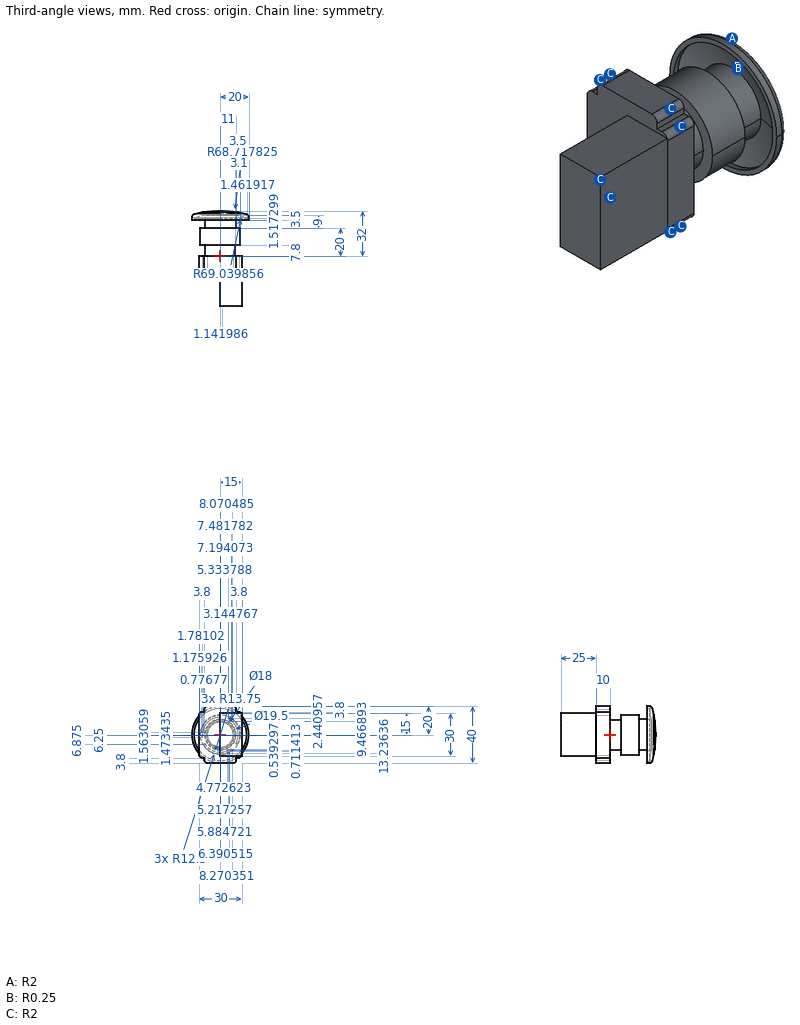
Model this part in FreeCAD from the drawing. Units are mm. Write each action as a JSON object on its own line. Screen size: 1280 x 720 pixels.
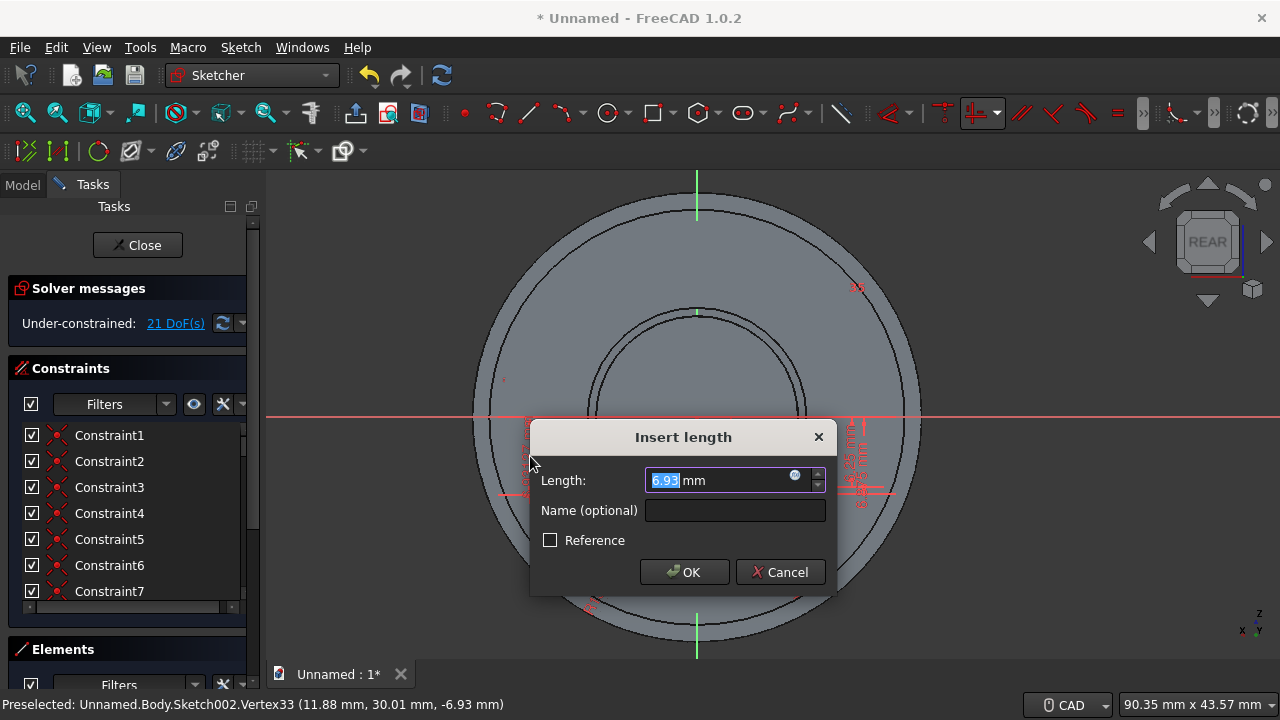
{"action": "type", "text": "6.875"}
{"action": "key", "text": "Return"}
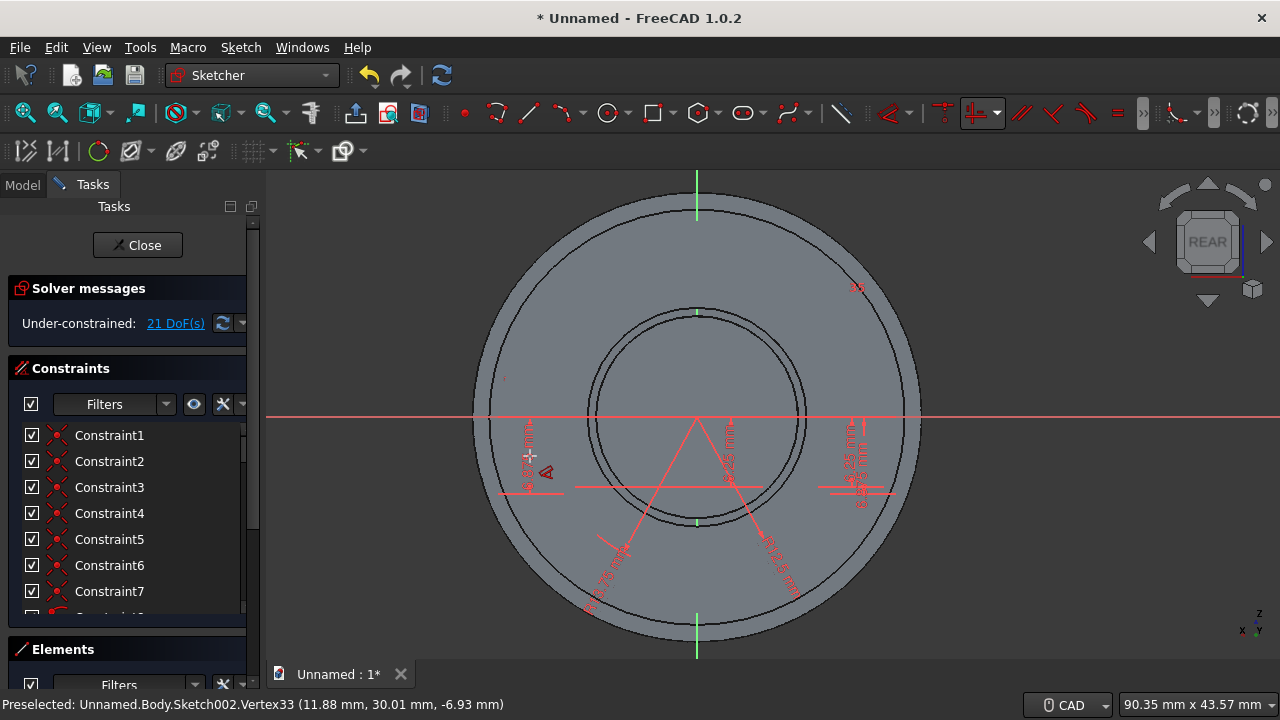
{"action": "scroll", "coordinate": [832, 401], "scroll_direction": "up", "scroll_amount": 8}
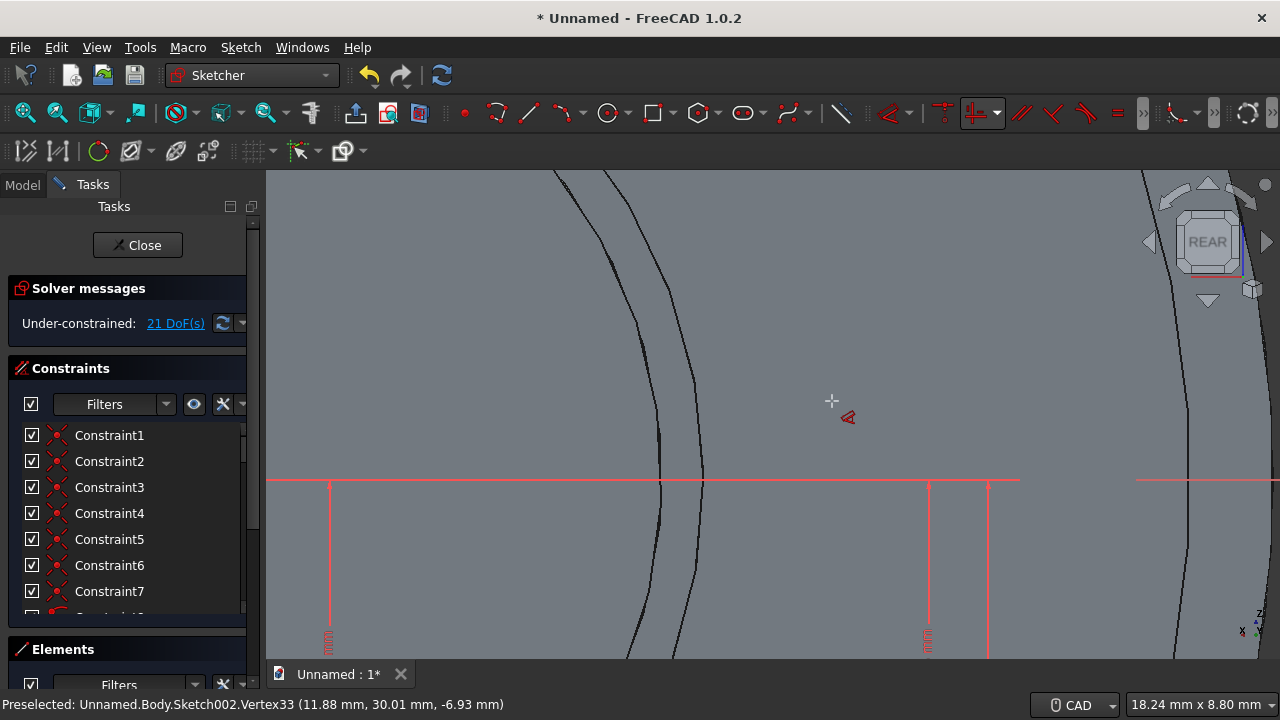
{"action": "left_click", "coordinate": [829, 397]}
{"action": "left_click", "coordinate": [829, 363]}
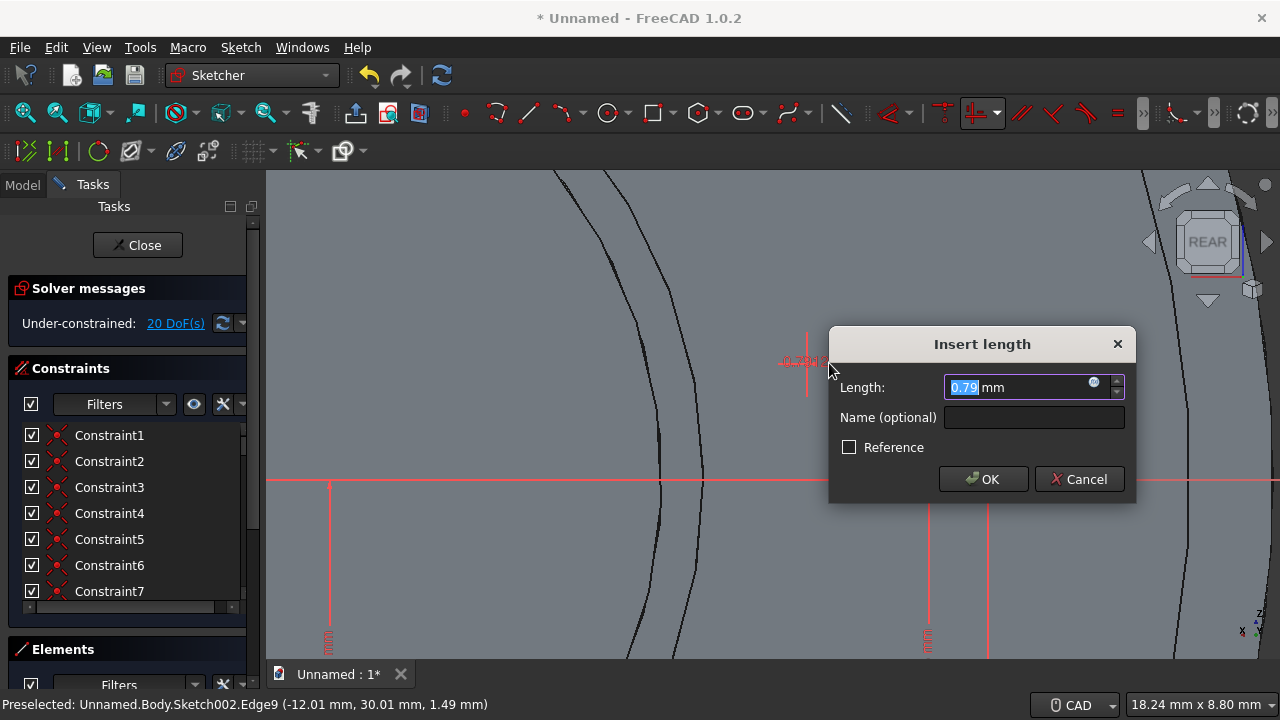
{"action": "type", "text": "0.77677"}
{"action": "key", "text": "Return"}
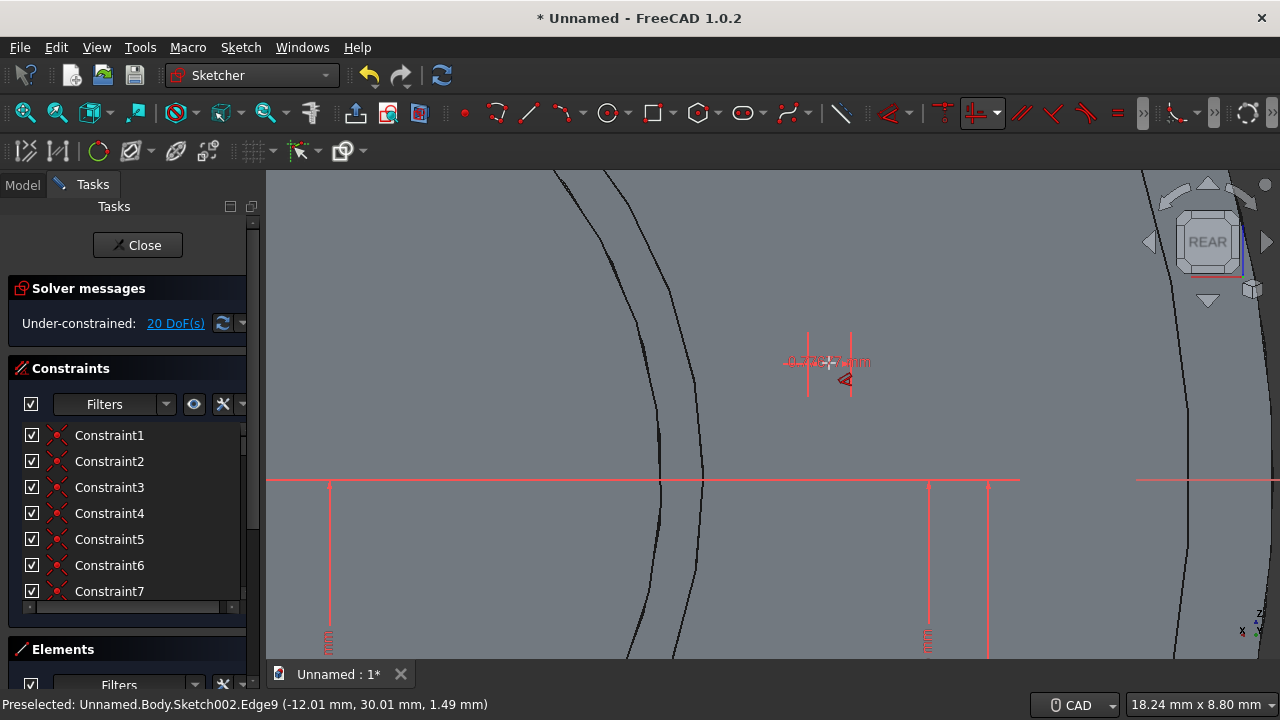
{"action": "left_click", "coordinate": [967, 396]}
{"action": "left_click", "coordinate": [954, 362]}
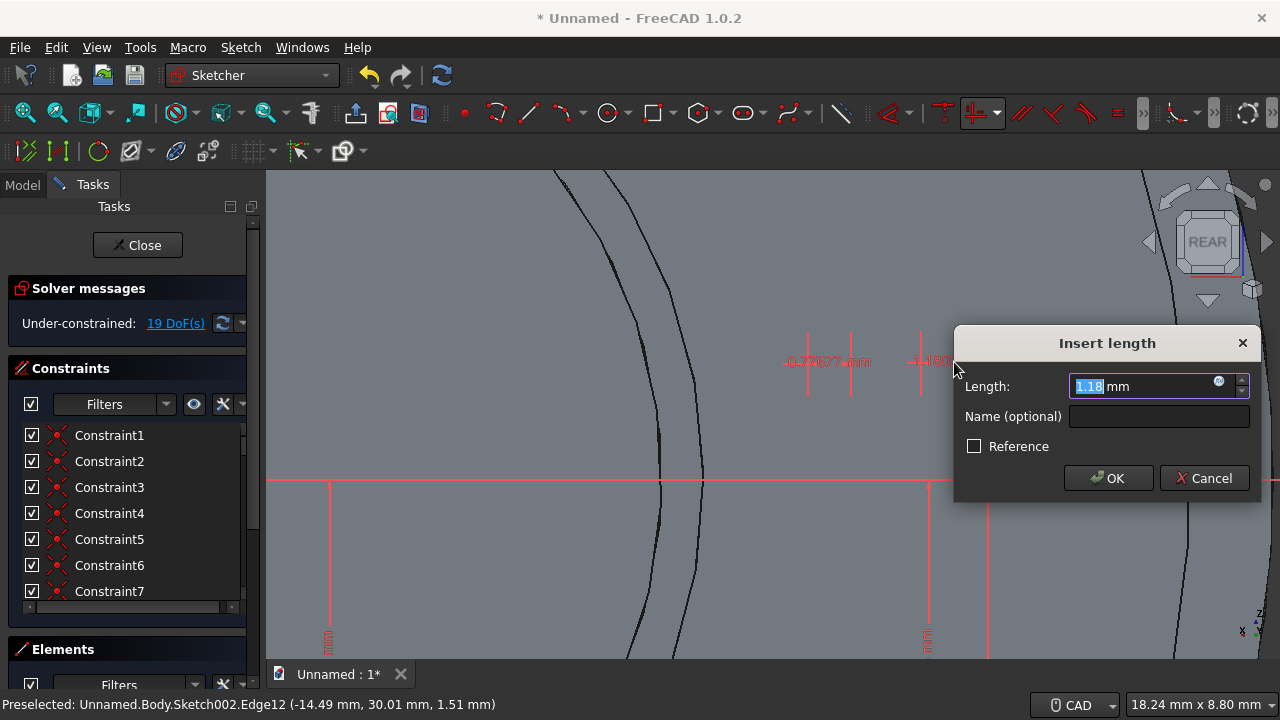
{"action": "type", "text": "1.175926"}
{"action": "key", "text": "Return"}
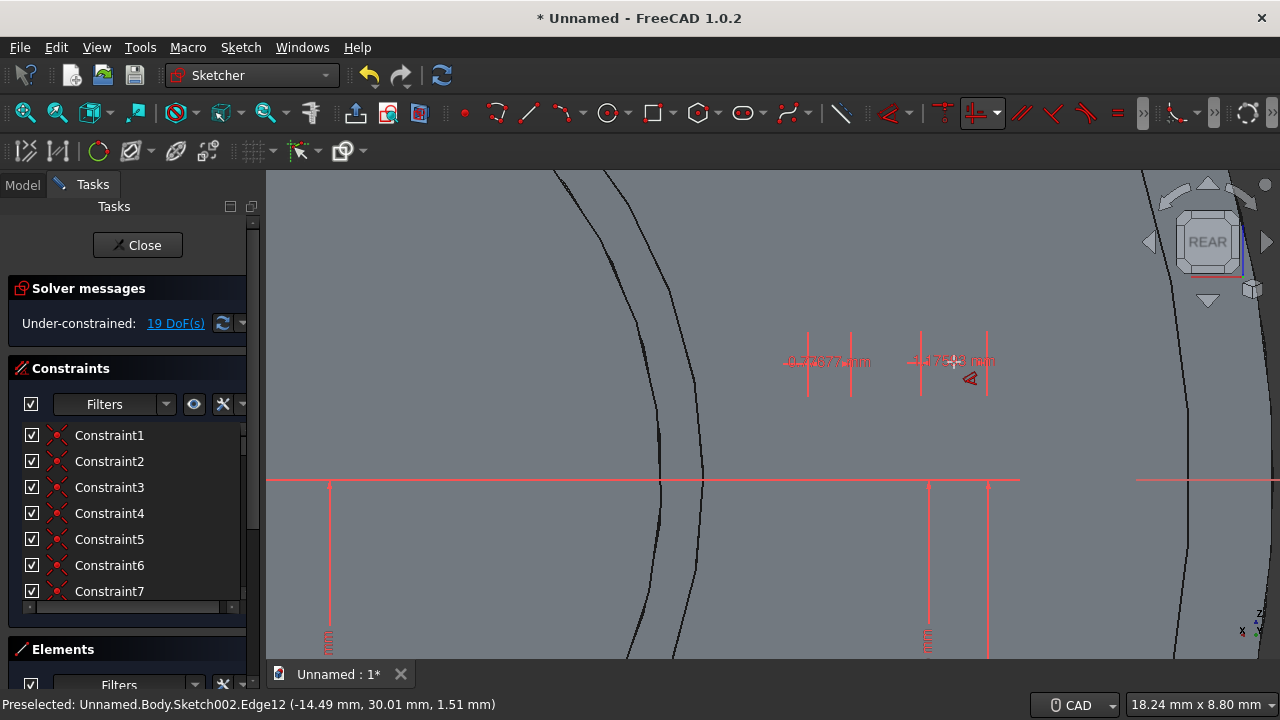
{"action": "scroll", "coordinate": [832, 402], "scroll_direction": "down", "scroll_amount": 8}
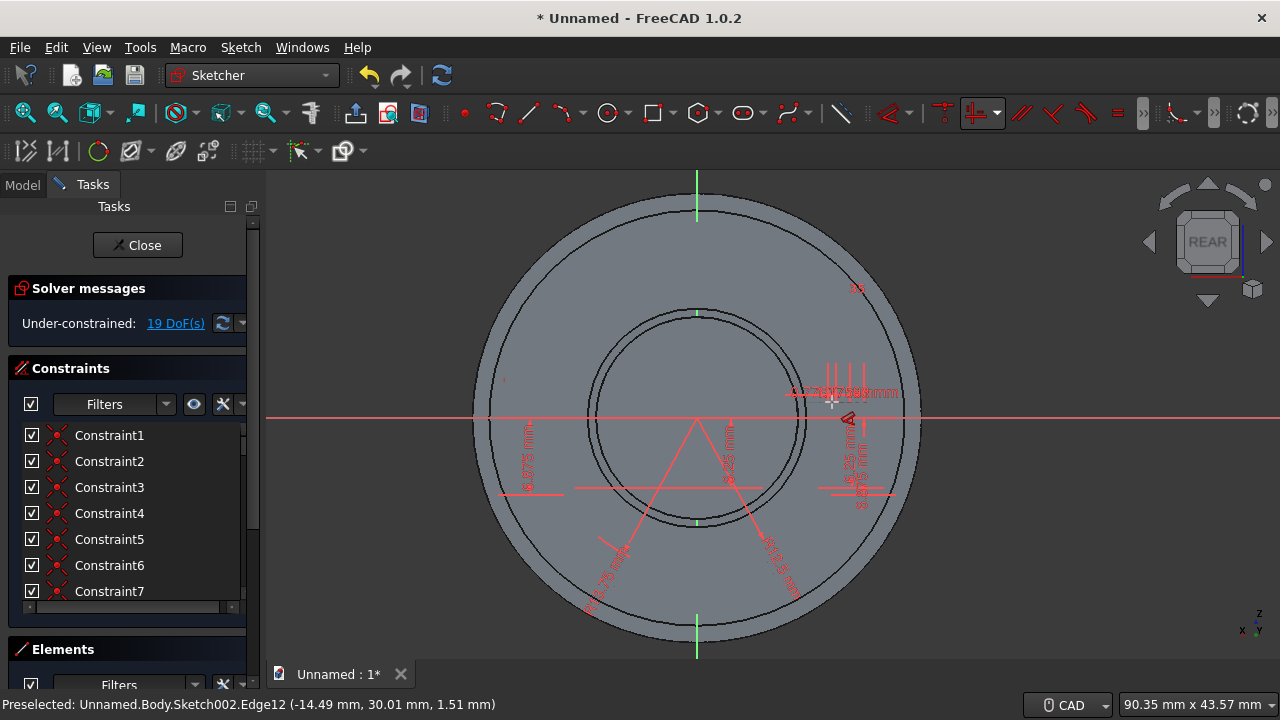
{"action": "scroll", "coordinate": [627, 285], "scroll_direction": "up", "scroll_amount": 3}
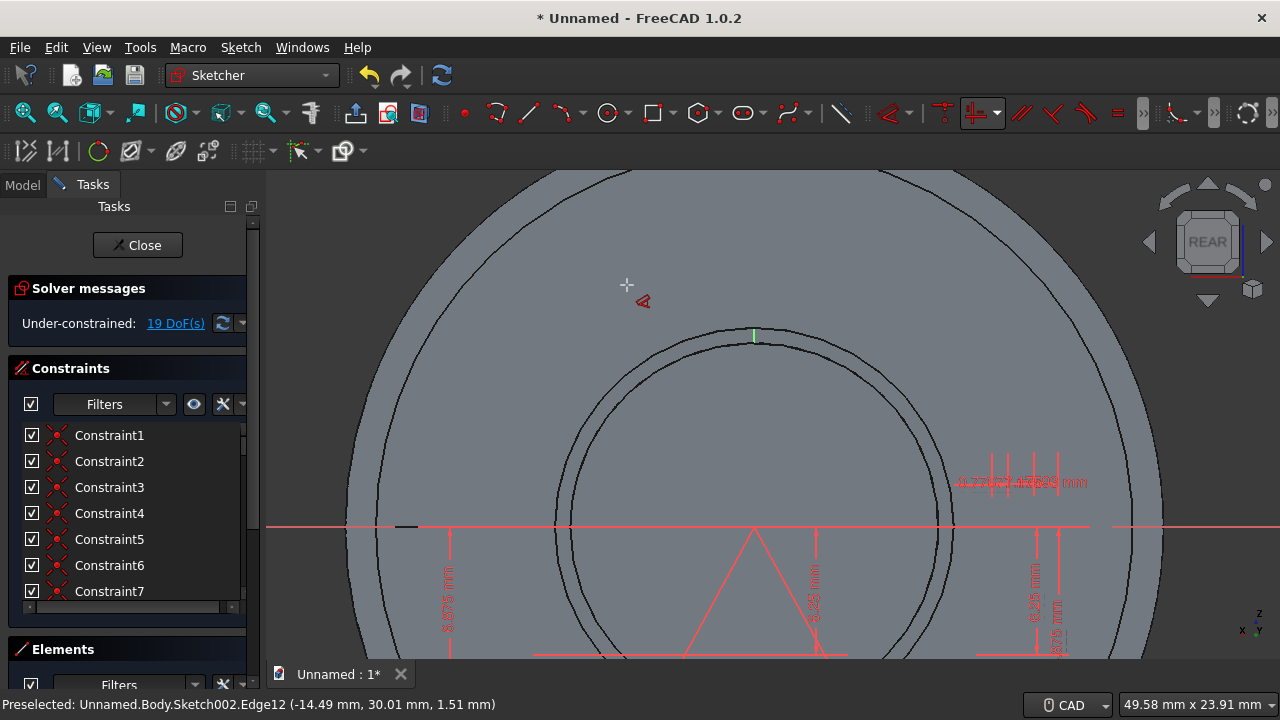
{"action": "left_click", "coordinate": [626, 284]}
{"action": "left_click", "coordinate": [613, 250]}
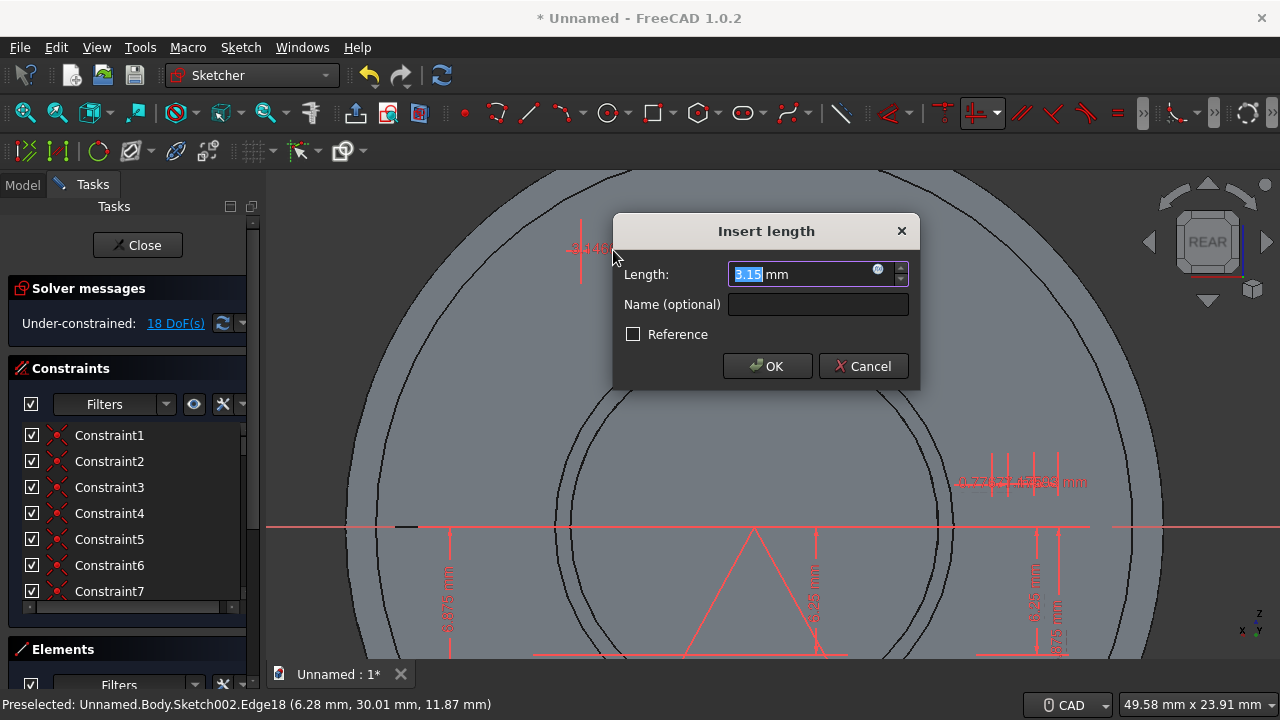
{"action": "type", "text": "3.144767"}
{"action": "key", "text": "Return"}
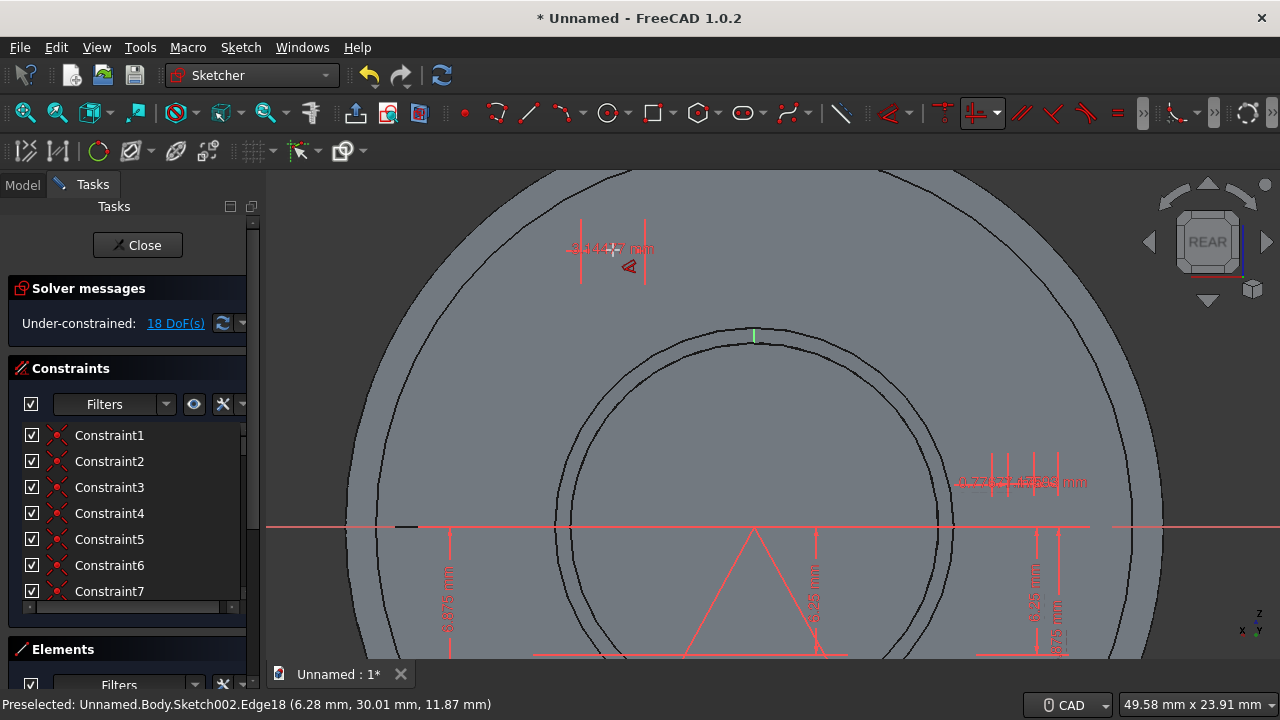
{"action": "left_click", "coordinate": [1032, 540]}
{"action": "left_click", "coordinate": [1048, 462]}